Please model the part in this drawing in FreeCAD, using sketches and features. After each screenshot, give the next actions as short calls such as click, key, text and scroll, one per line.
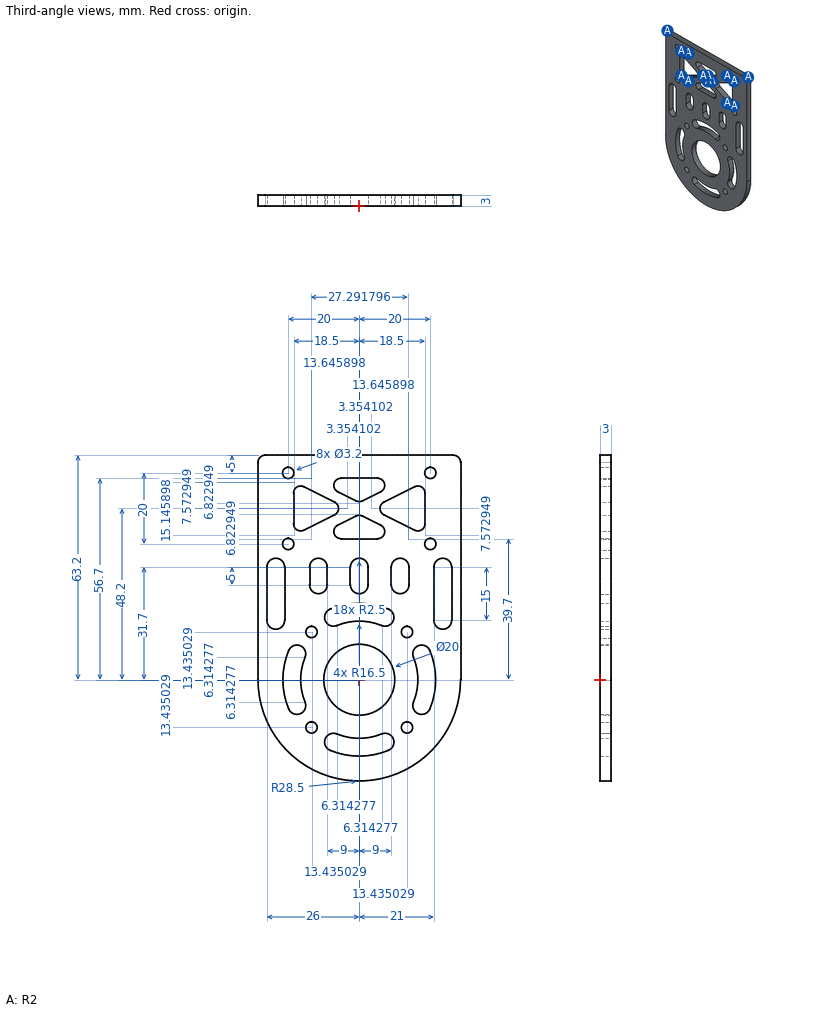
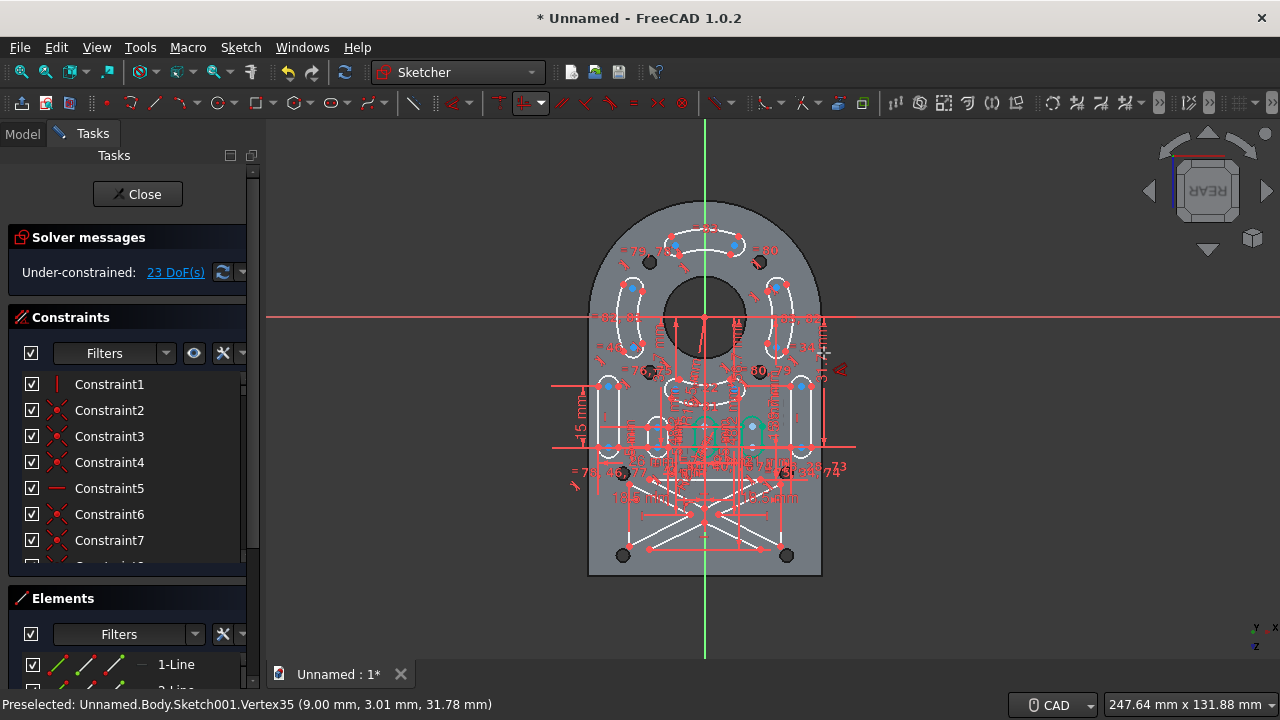
click(791, 448)
click(849, 383)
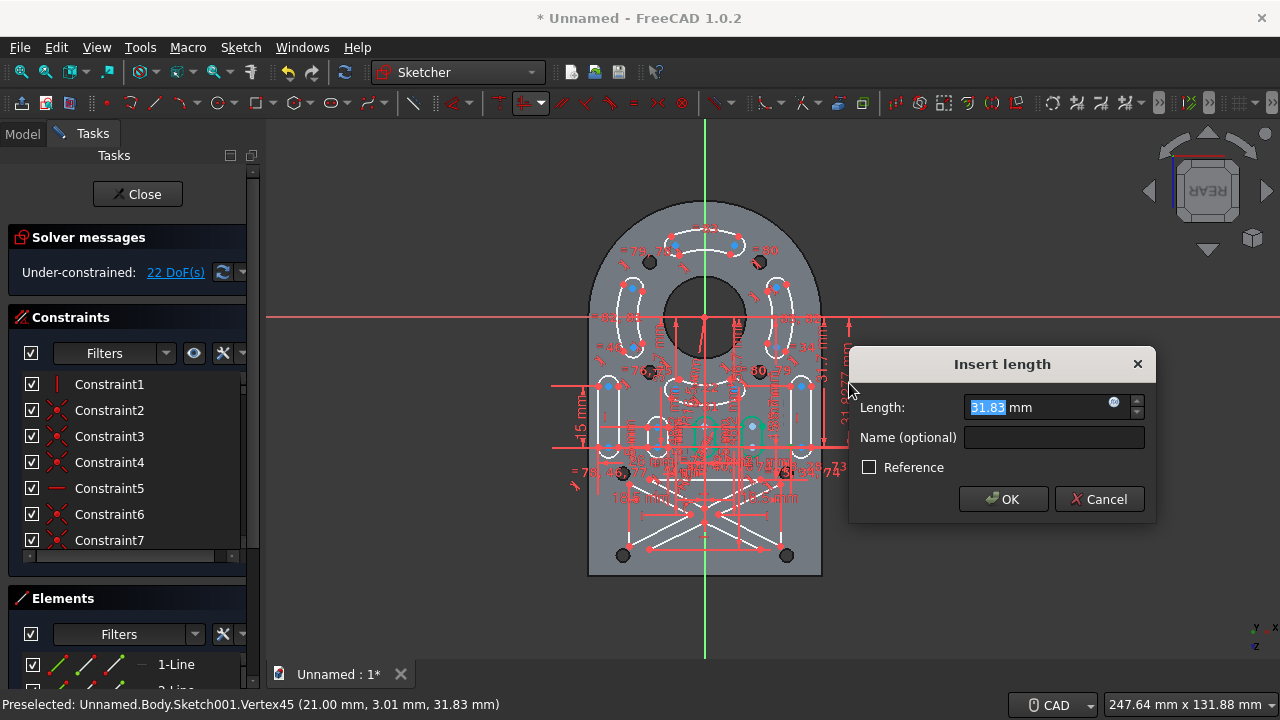
text(31.7)
key(Return)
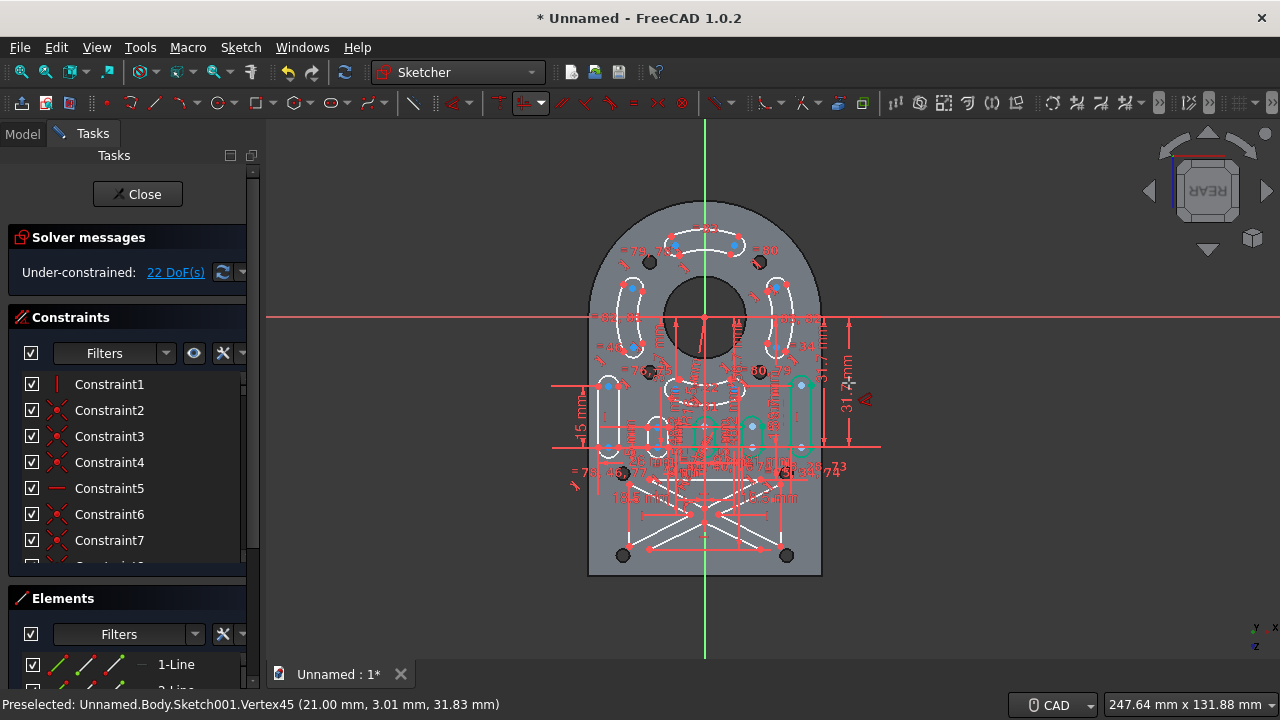
click(648, 448)
click(590, 353)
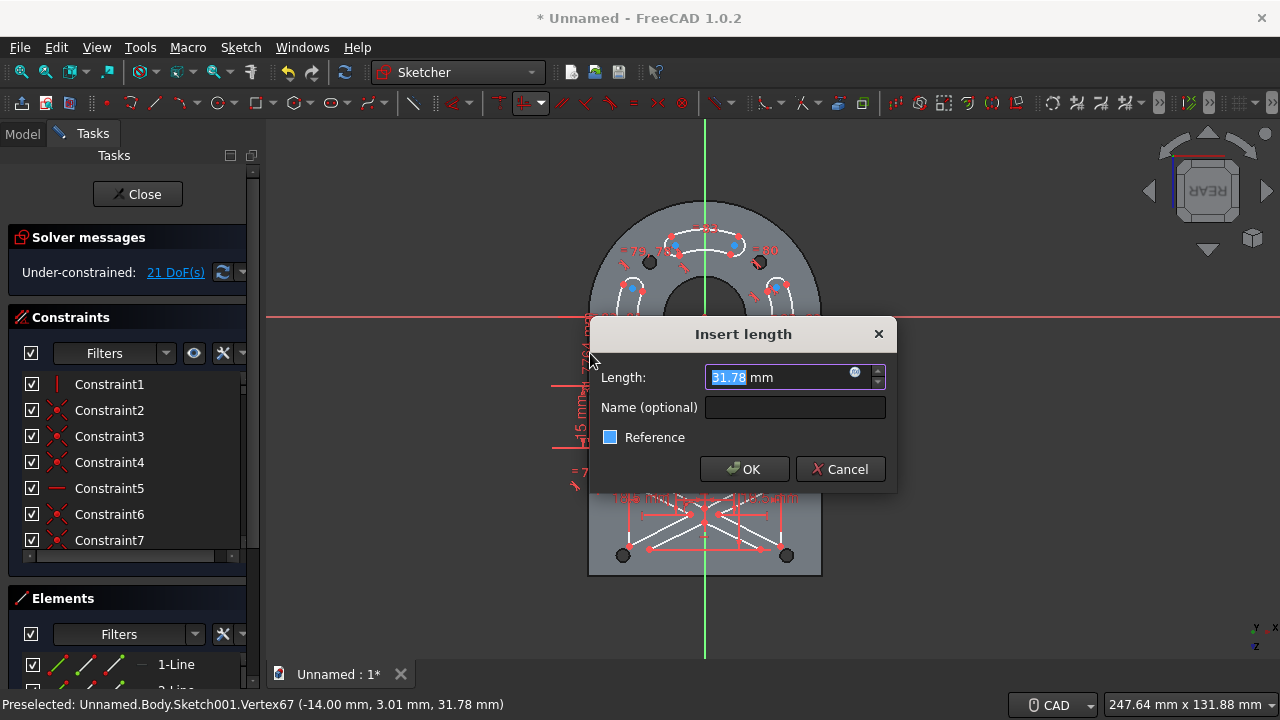
text(31.7)
key(Return)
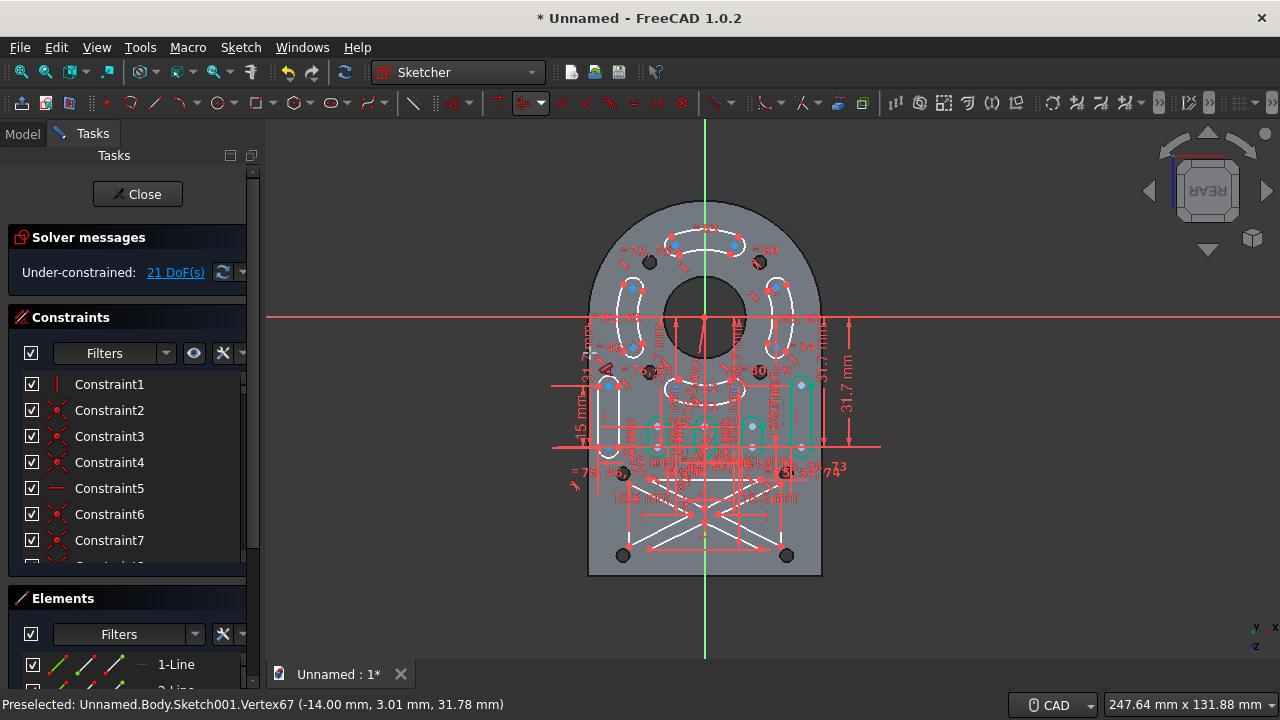
click(598, 448)
click(564, 382)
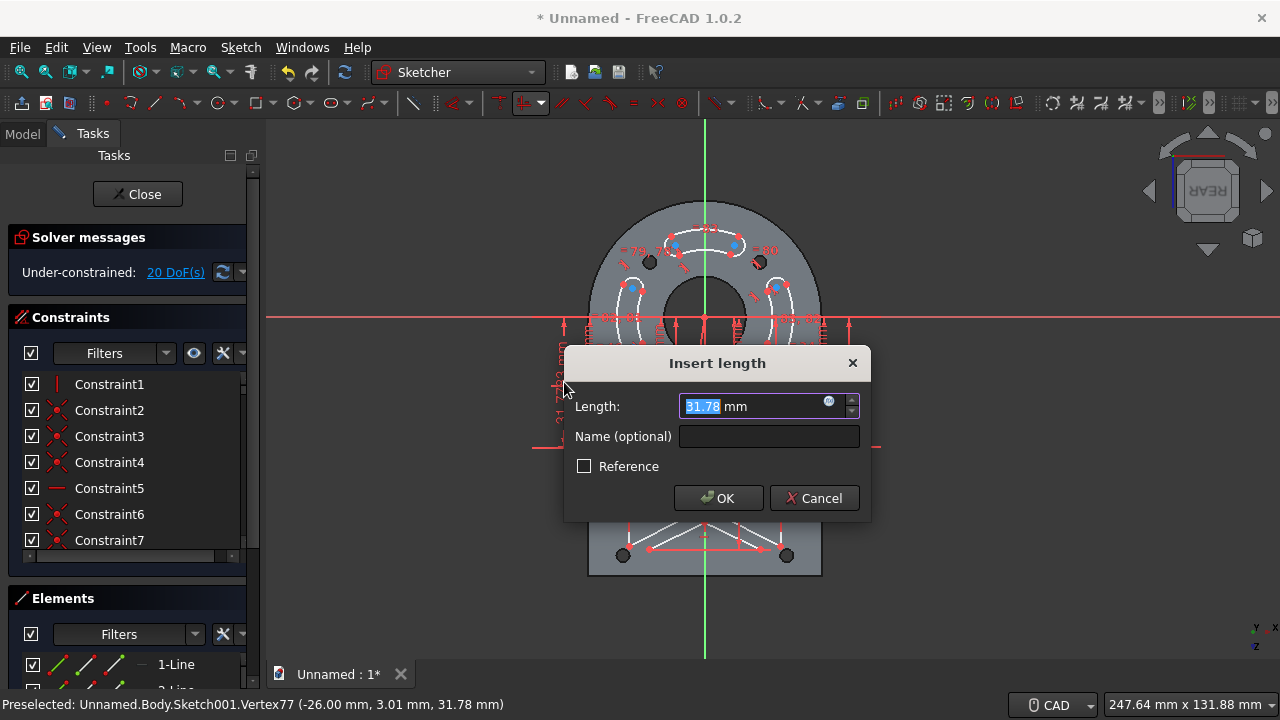
text(31.7)
key(Return)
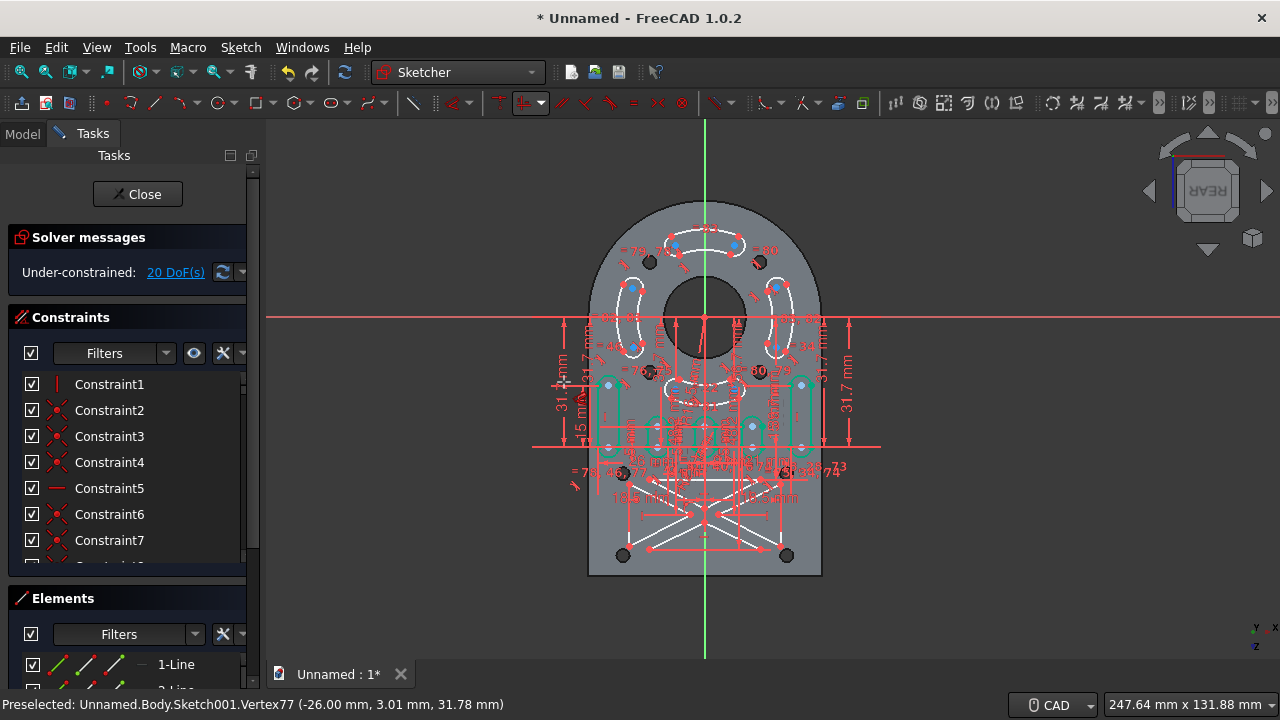
click(629, 503)
click(595, 530)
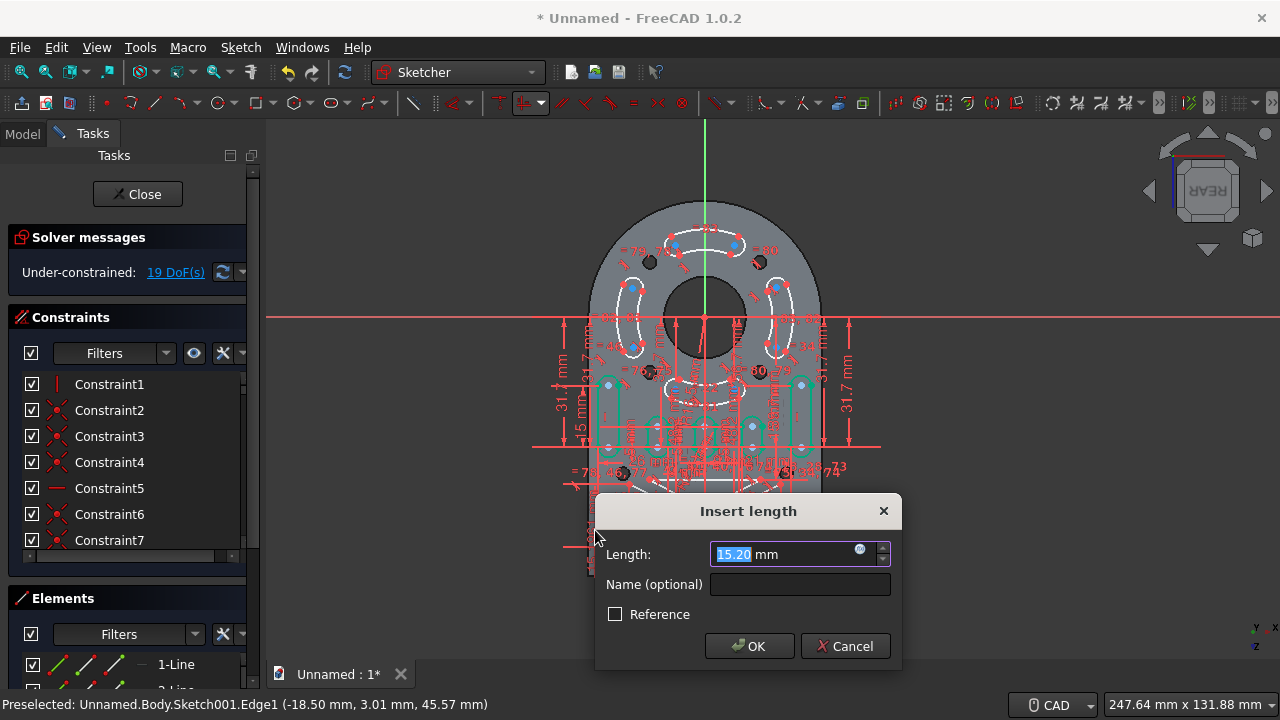
text(15.145898)
key(Return)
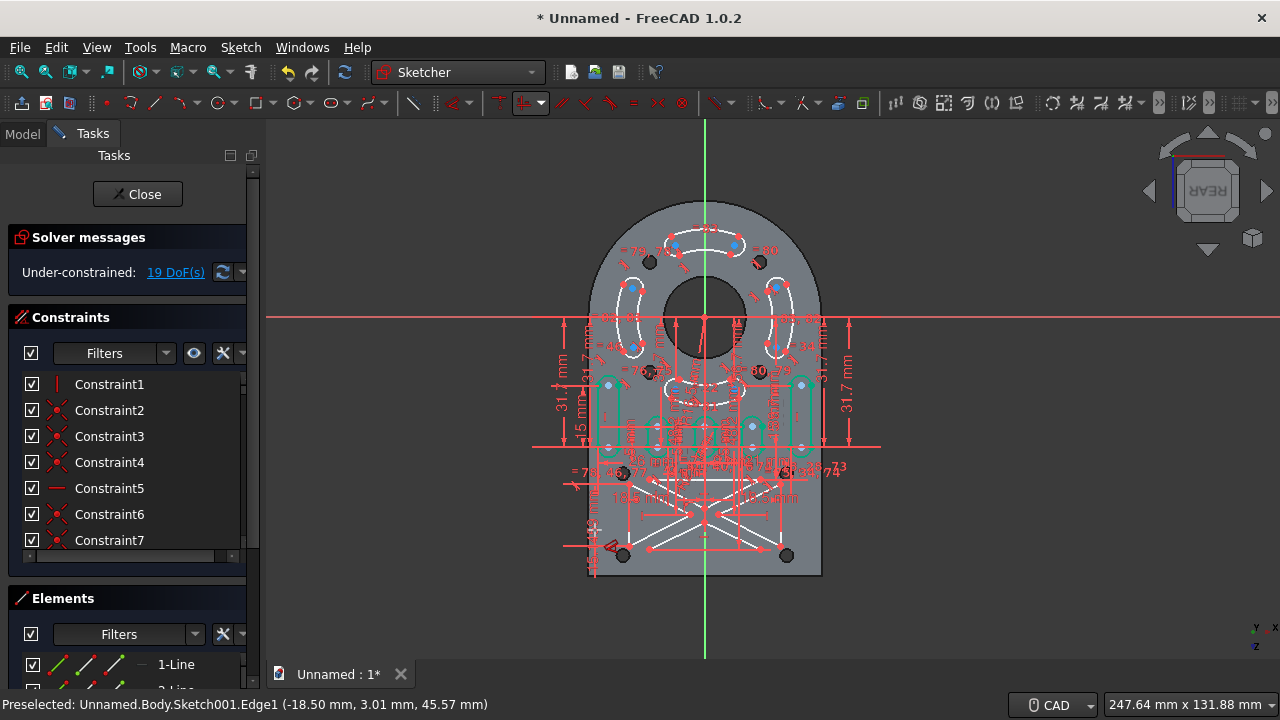
click(727, 480)
click(679, 586)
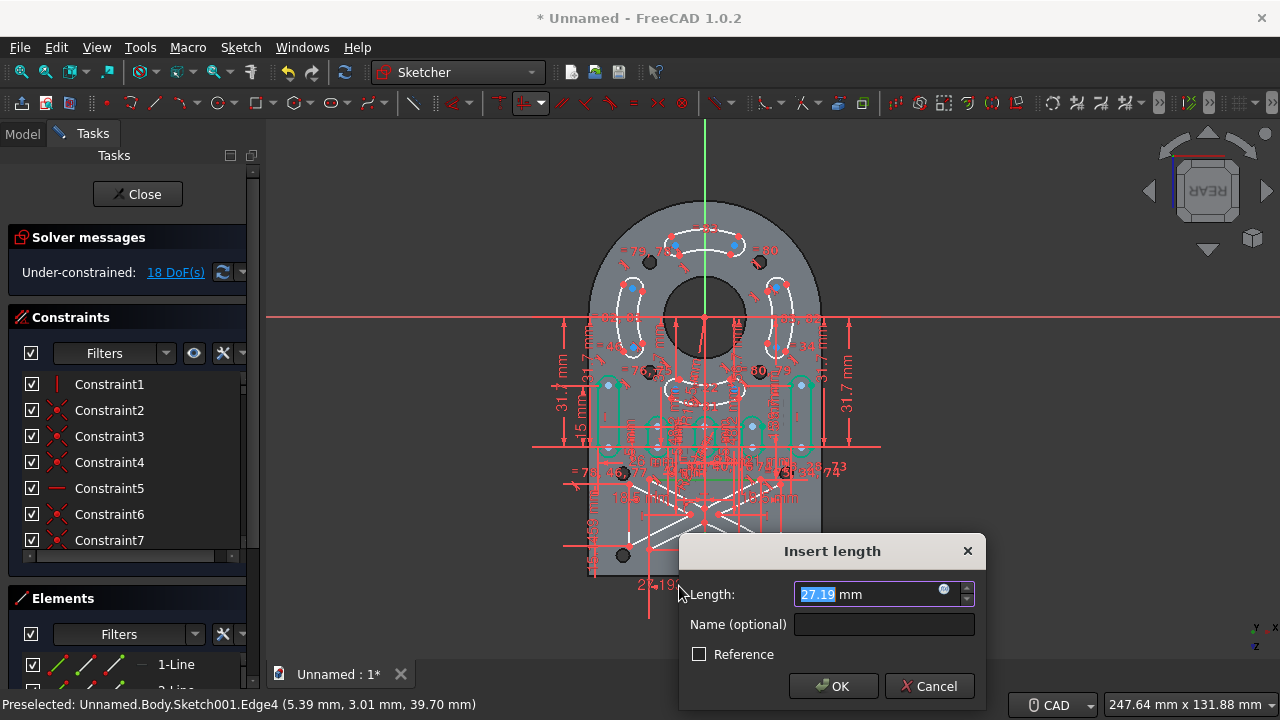
text(27.291796)
key(Return)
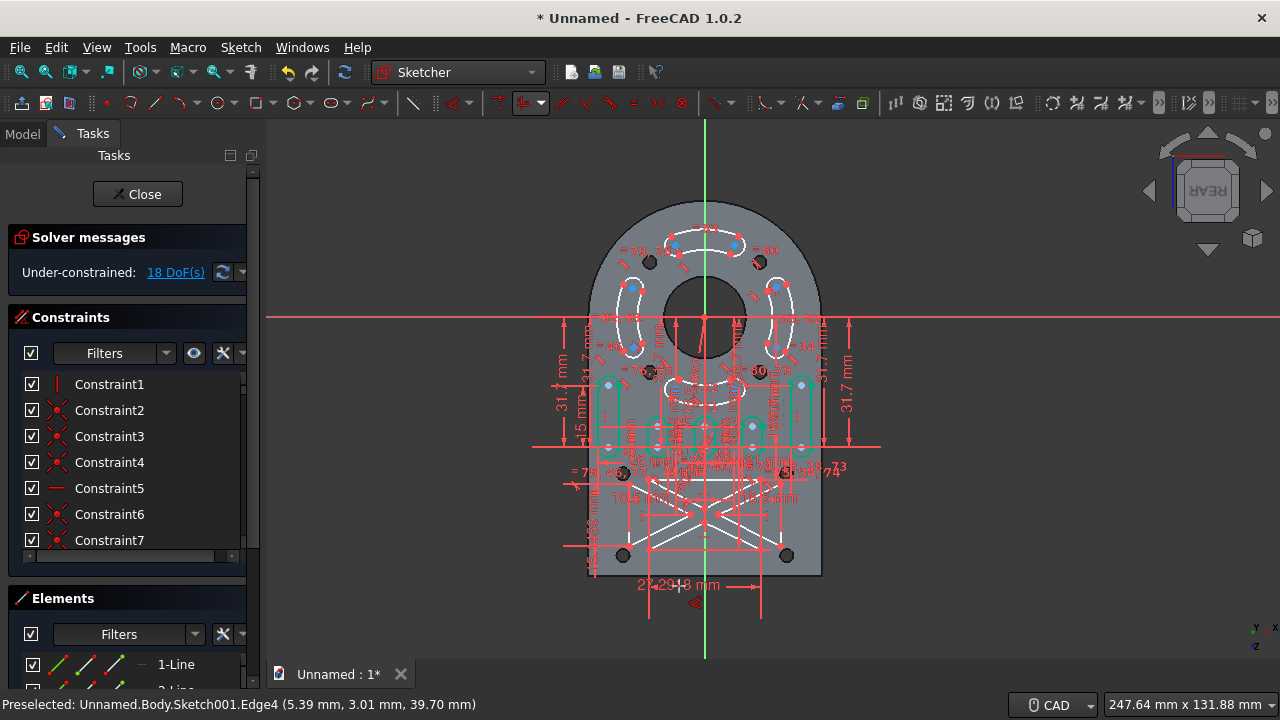
click(781, 528)
click(815, 530)